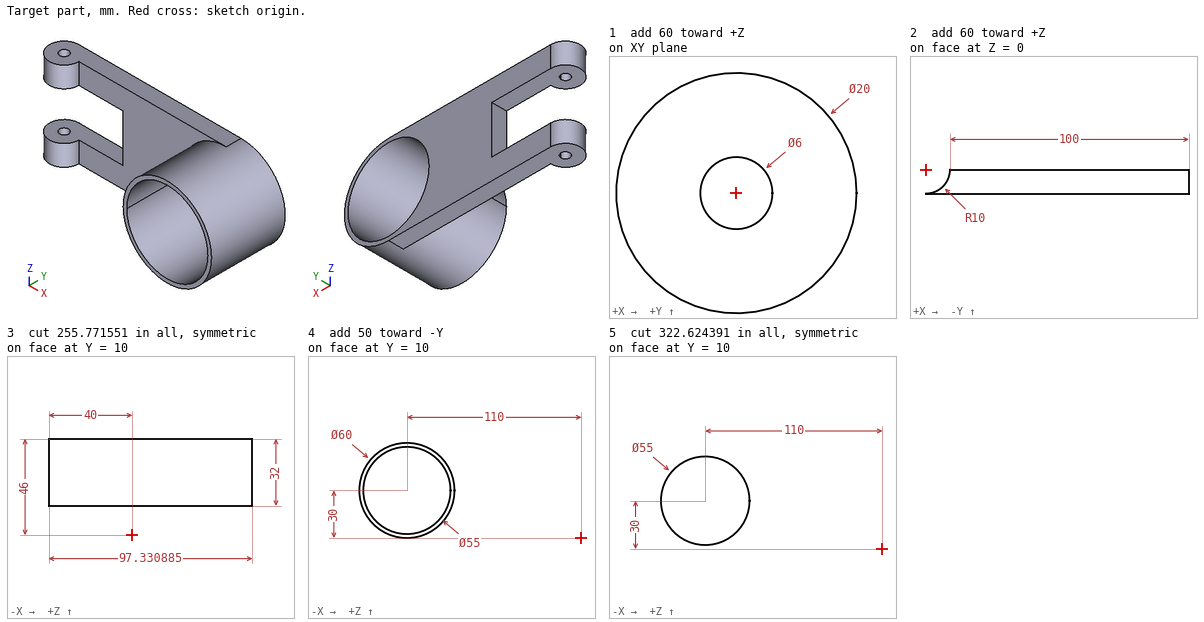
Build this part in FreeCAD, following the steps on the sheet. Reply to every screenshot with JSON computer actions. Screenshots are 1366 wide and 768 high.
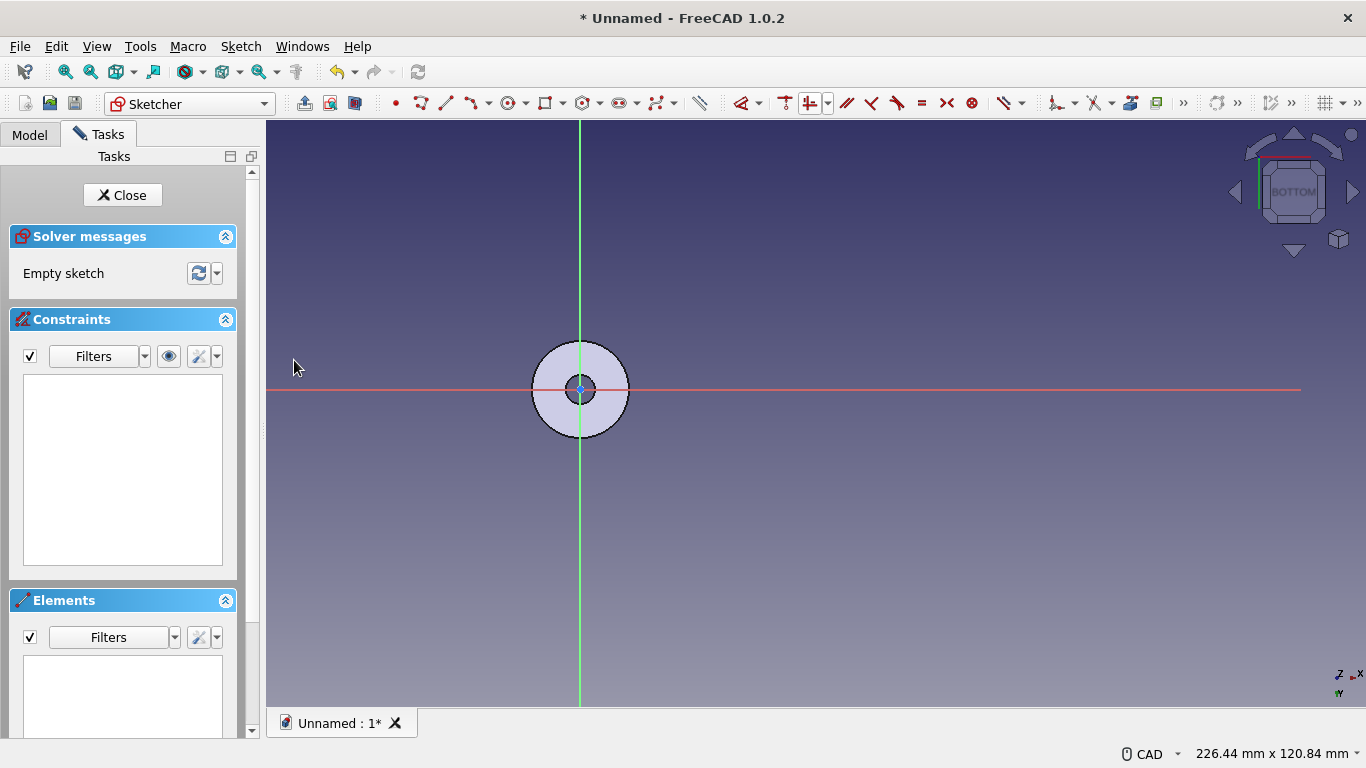
{"action": "left_click", "coordinate": [421, 104]}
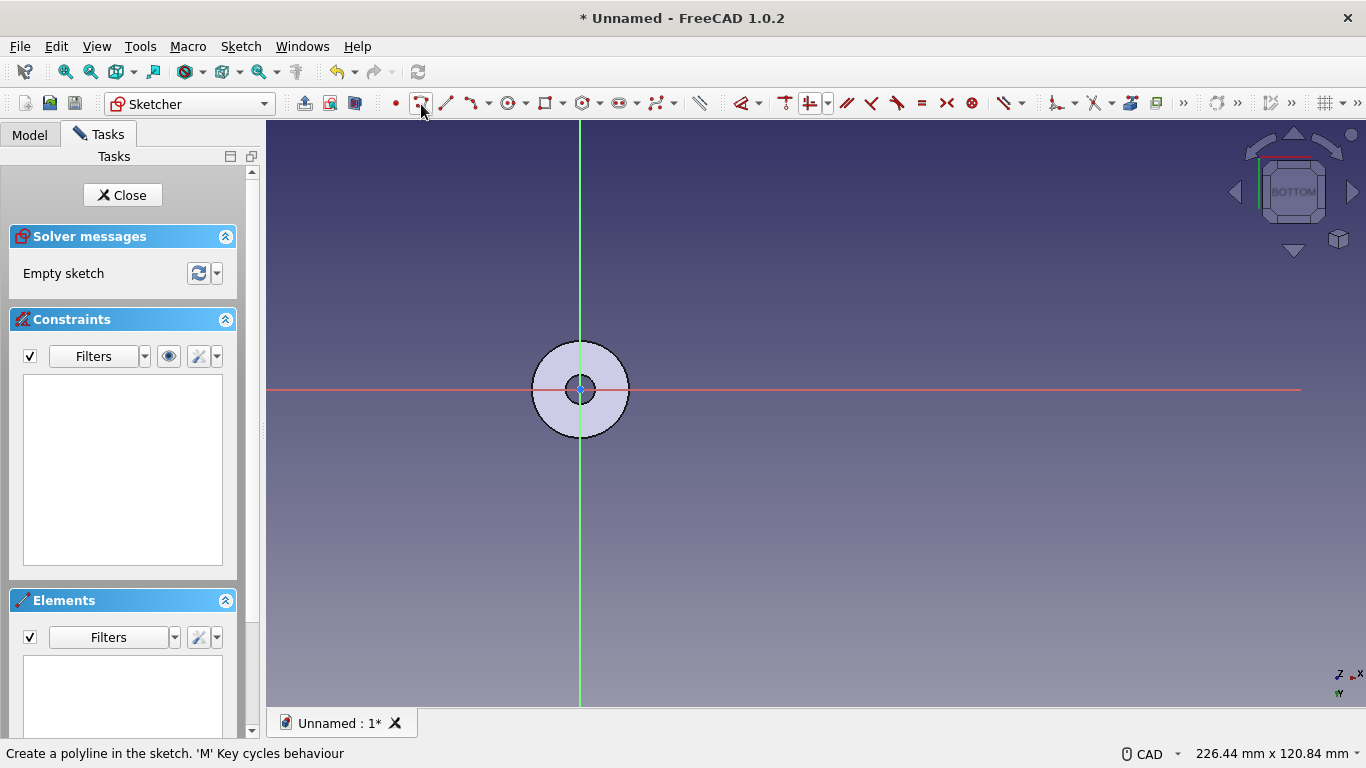
{"action": "left_click", "coordinate": [629, 390]}
{"action": "left_click", "coordinate": [1115, 399]}
{"action": "left_click", "coordinate": [1115, 438]}
{"action": "left_click", "coordinate": [580, 438]}
{"action": "right_click", "coordinate": [580, 438]}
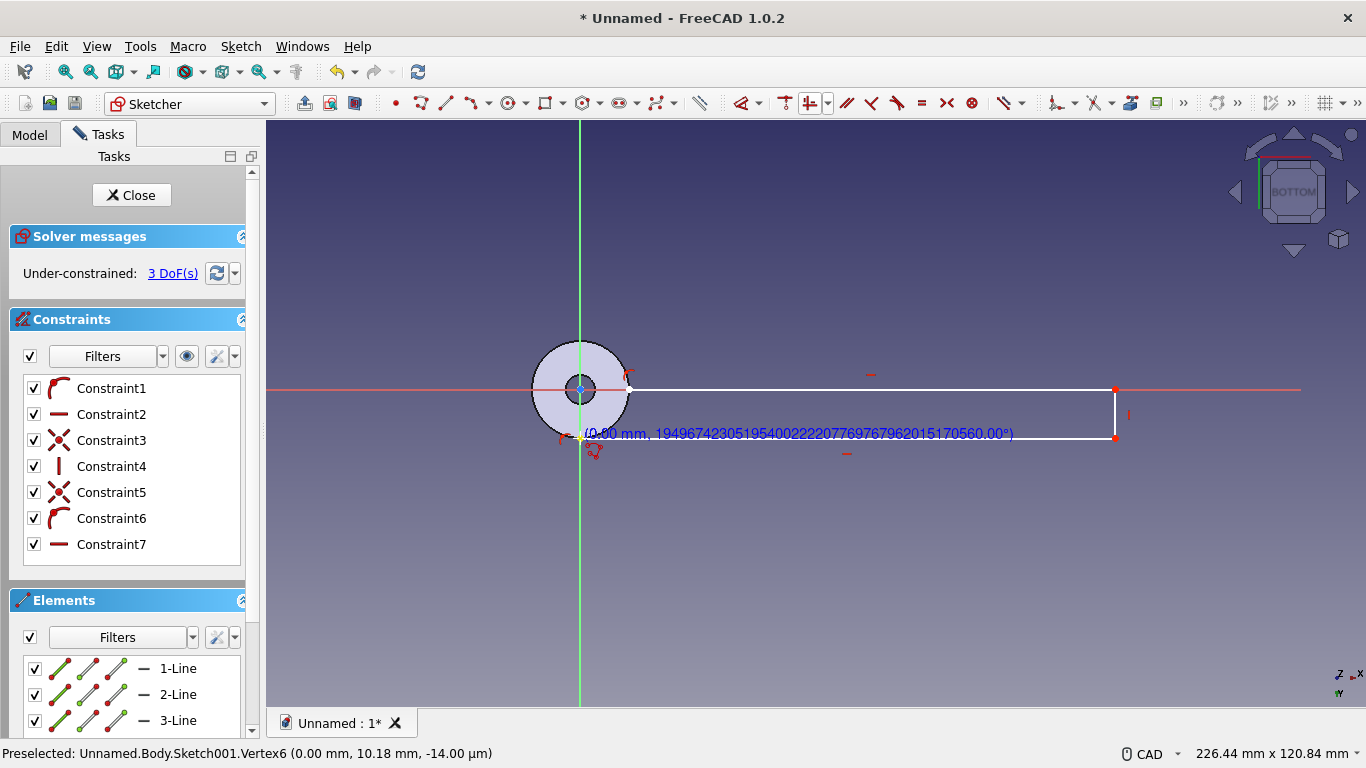
{"action": "left_click", "coordinate": [470, 104]}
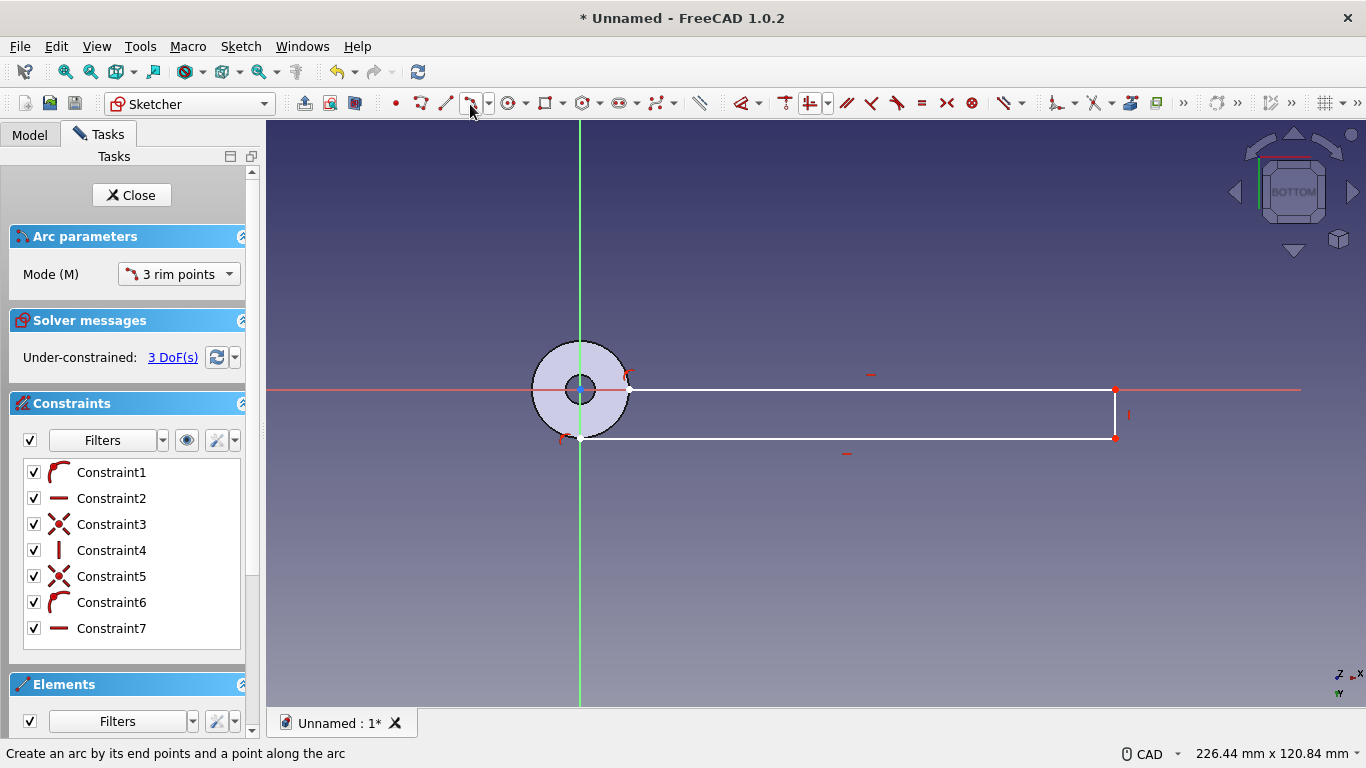
{"action": "left_click", "coordinate": [580, 439]}
{"action": "left_click", "coordinate": [629, 390]}
{"action": "left_click", "coordinate": [615, 424]}
{"action": "key", "text": "Escape"}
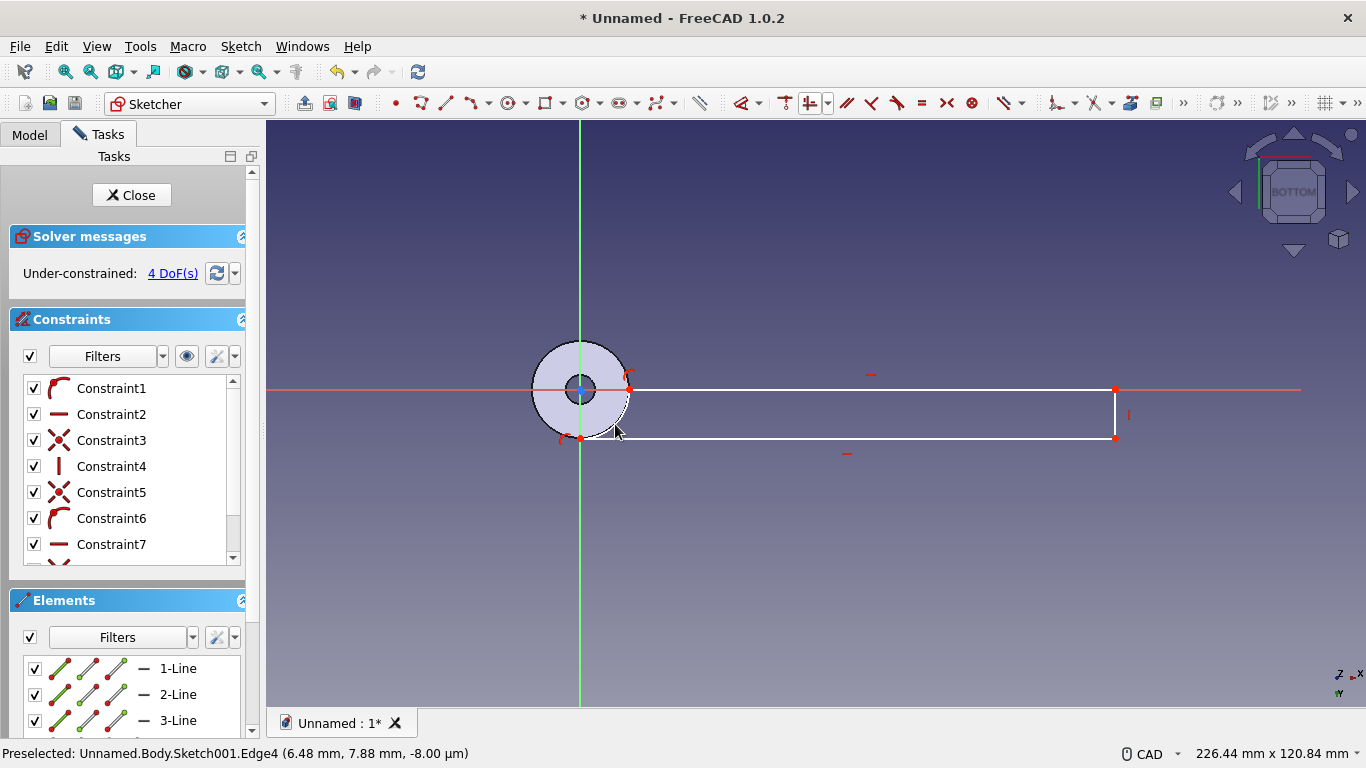
{"action": "left_click", "coordinate": [955, 439]}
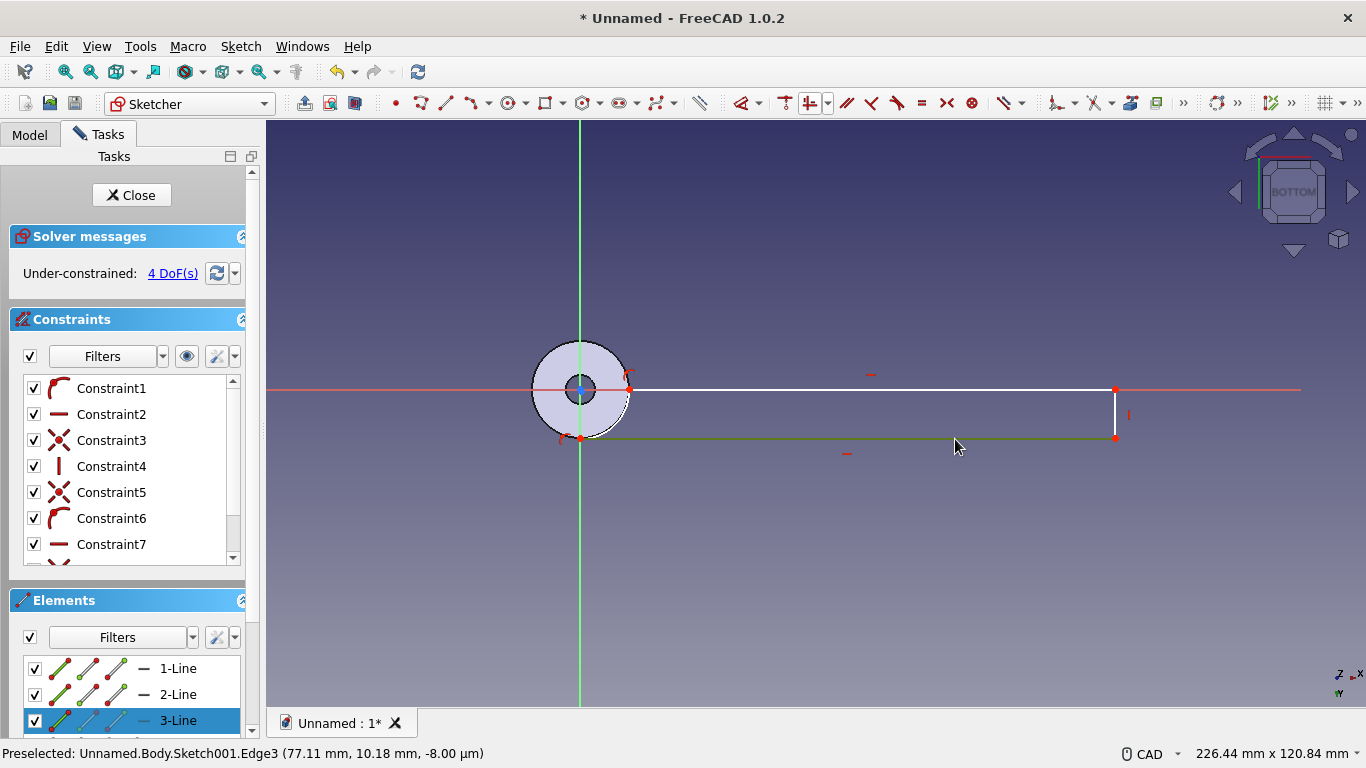
{"action": "left_click", "coordinate": [624, 412]}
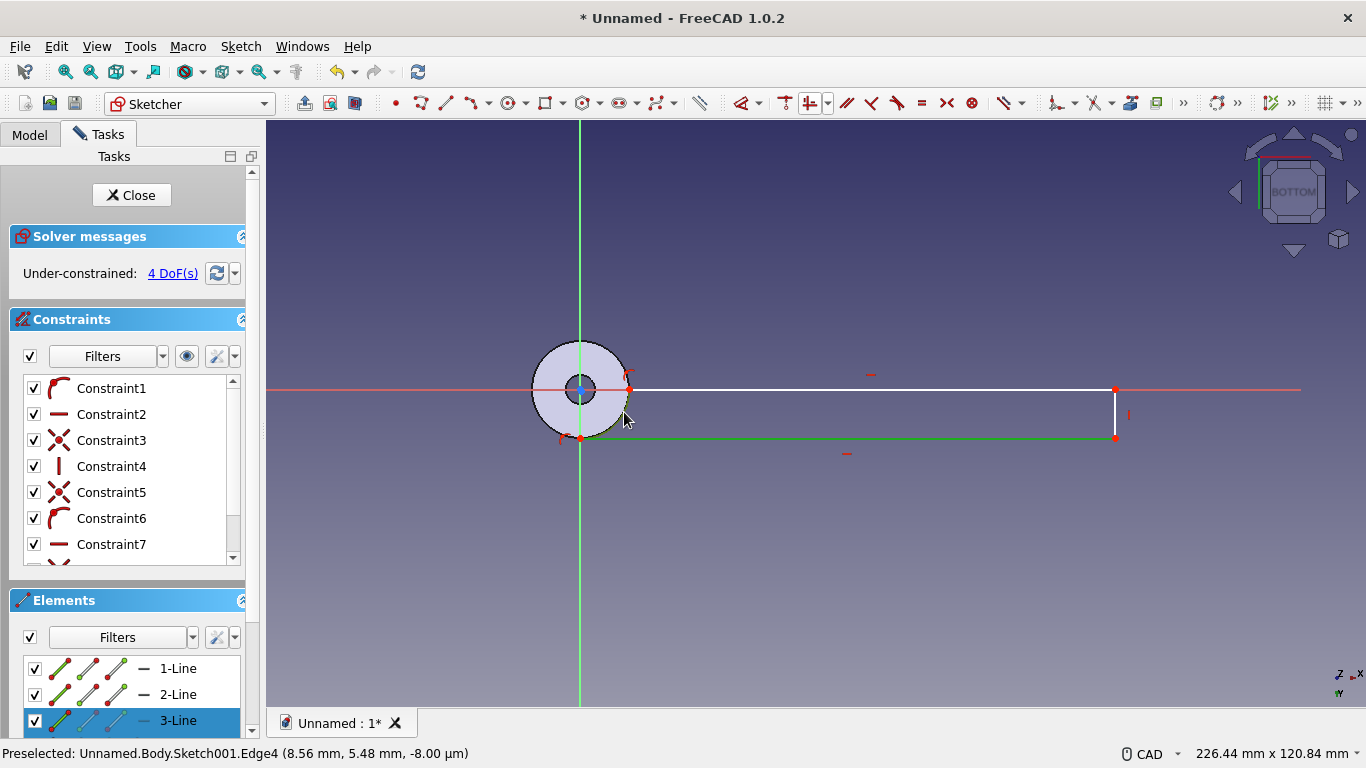
{"action": "left_click", "coordinate": [897, 104]}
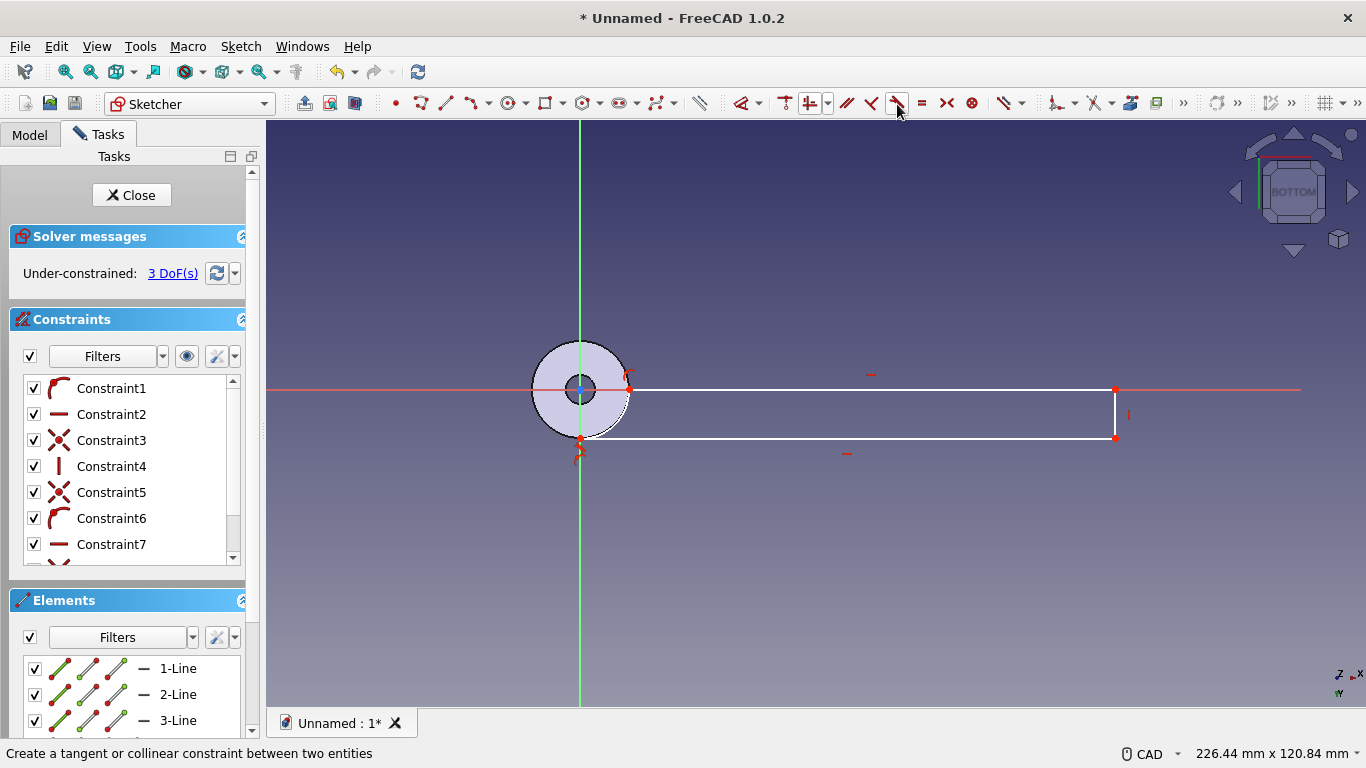
{"action": "left_click", "coordinate": [580, 390]}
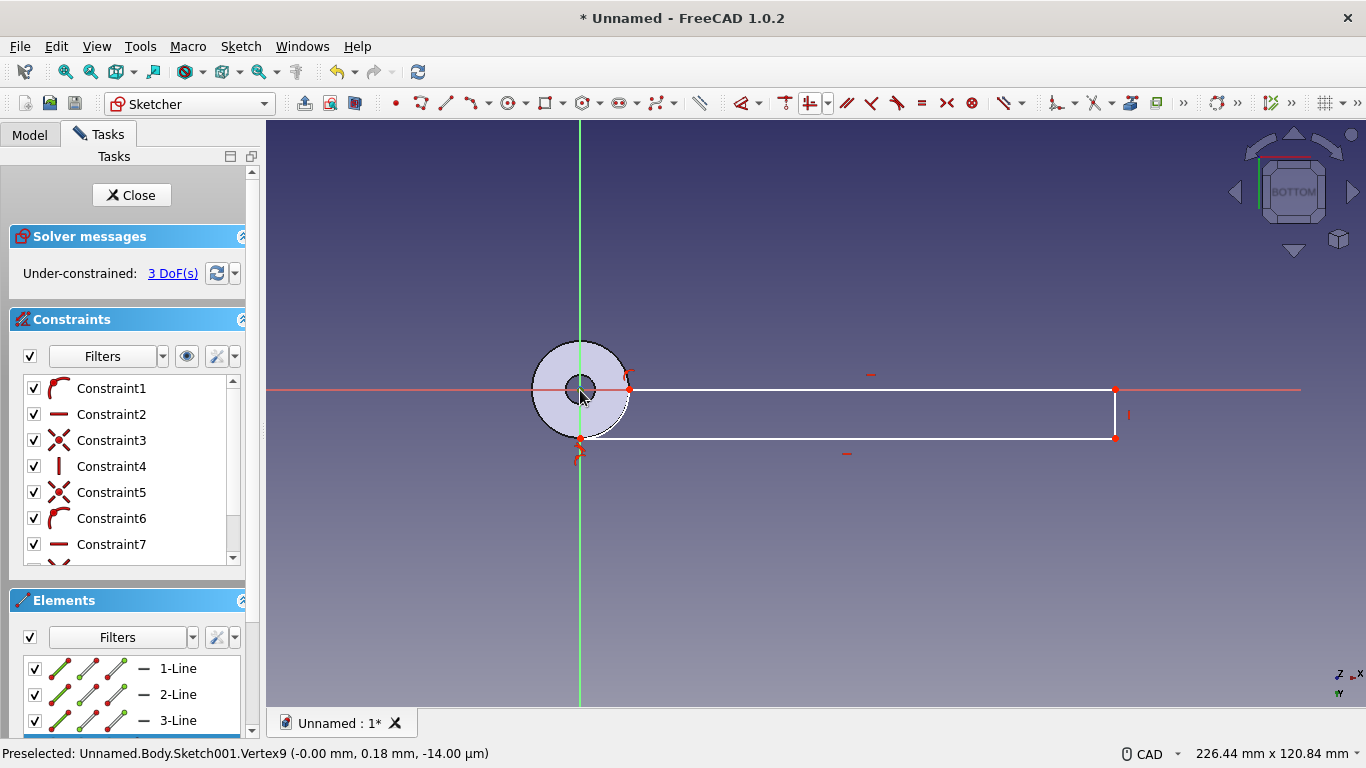
{"action": "left_click", "coordinate": [359, 390]}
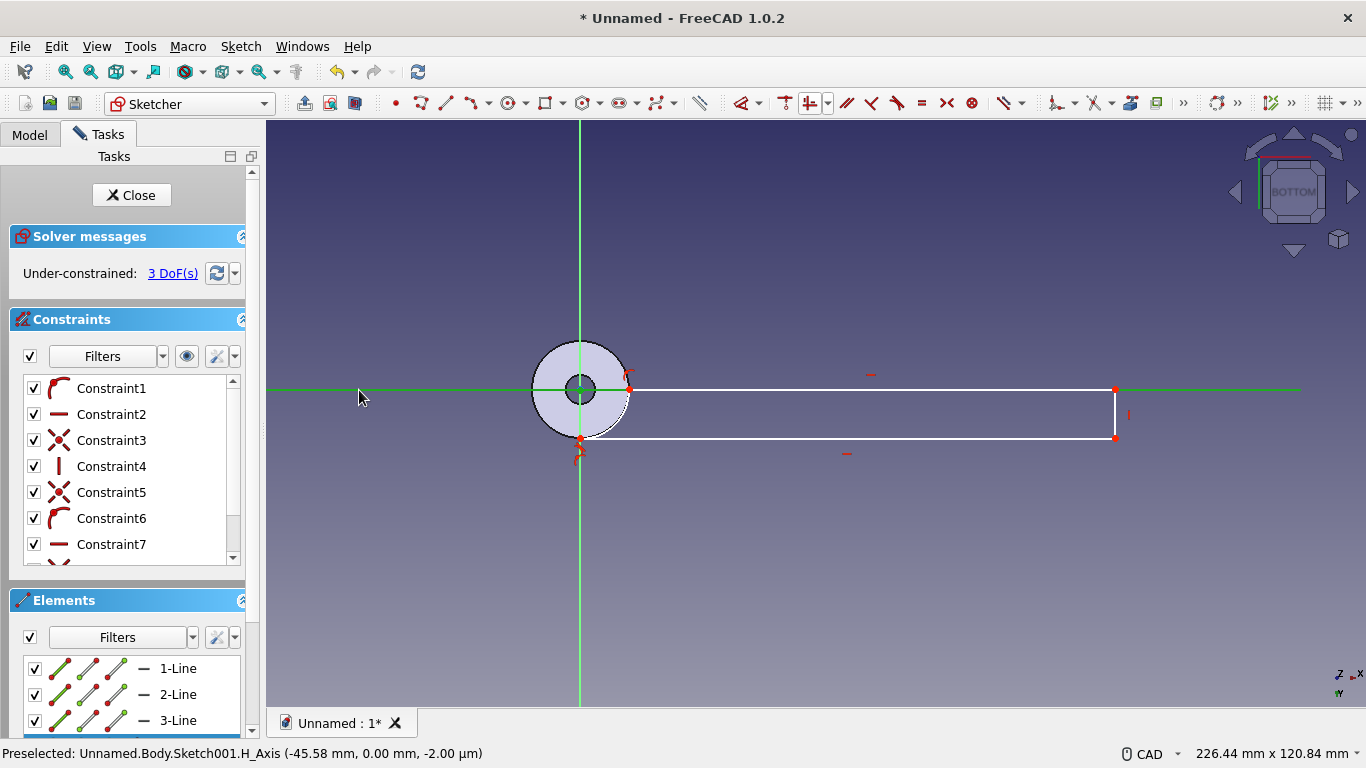
{"action": "left_click", "coordinate": [785, 104]}